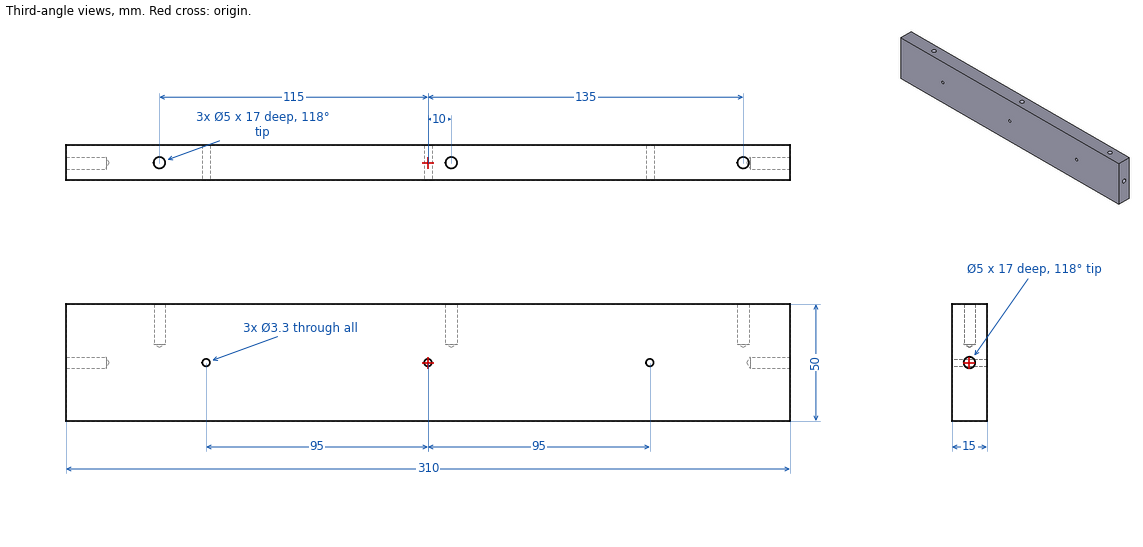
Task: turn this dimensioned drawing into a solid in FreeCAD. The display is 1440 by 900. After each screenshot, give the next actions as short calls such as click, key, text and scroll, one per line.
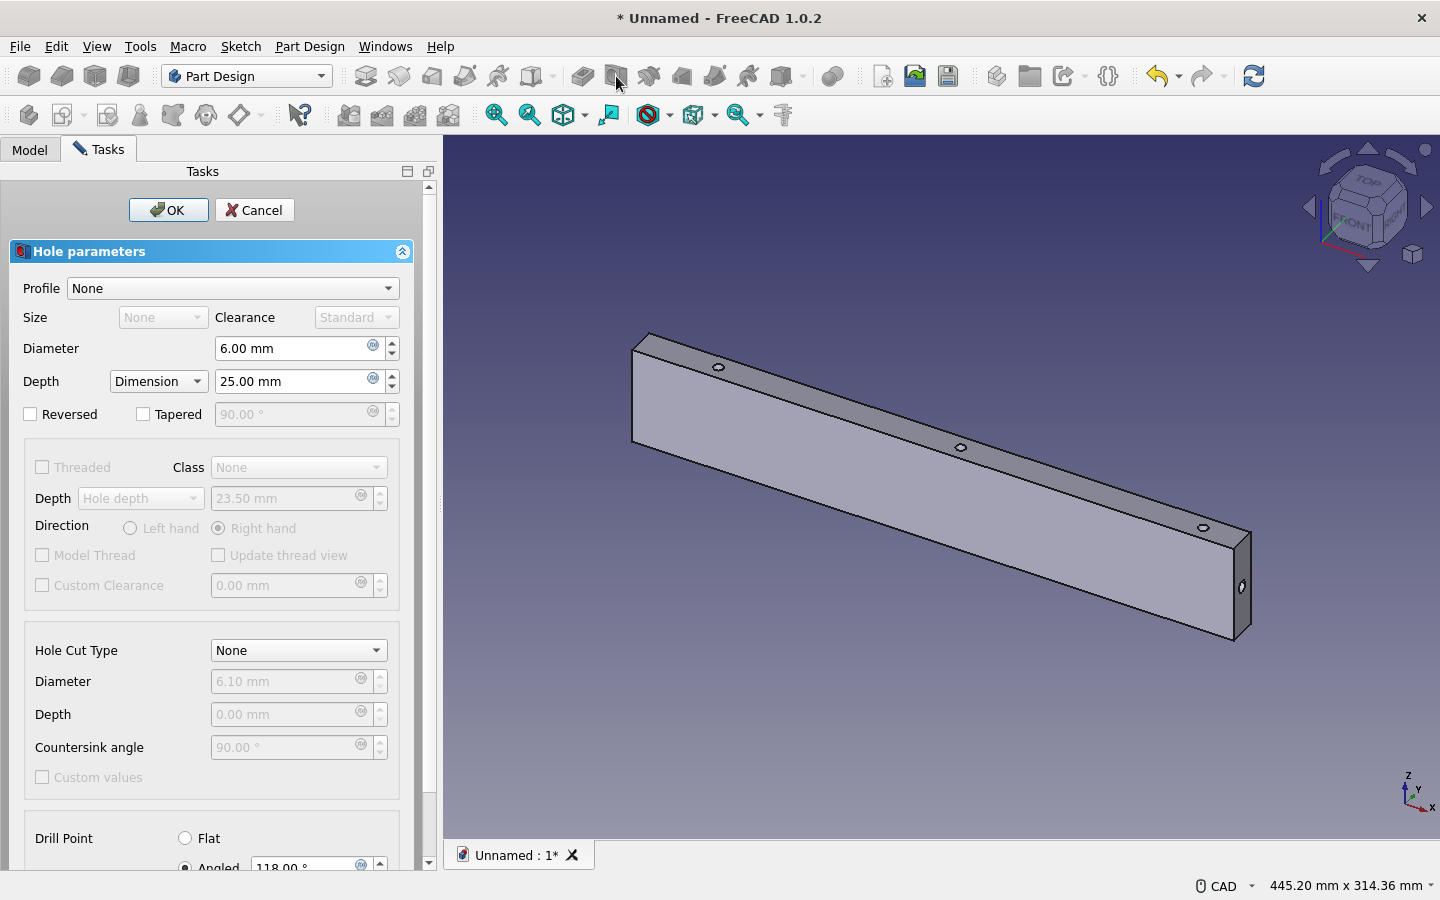
triple_click(300, 348)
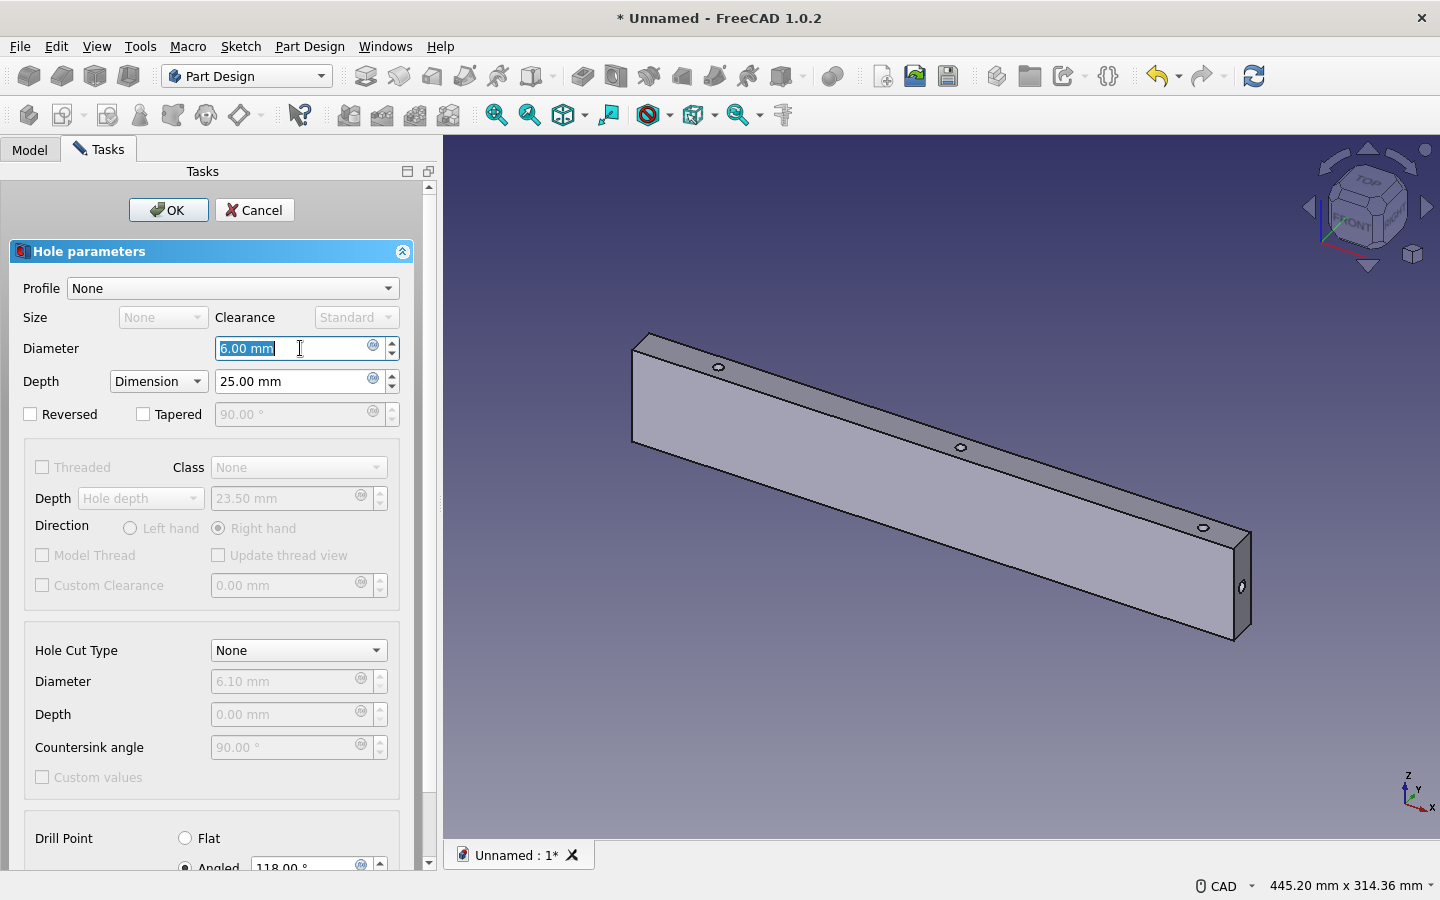
text(5)
key(Tab)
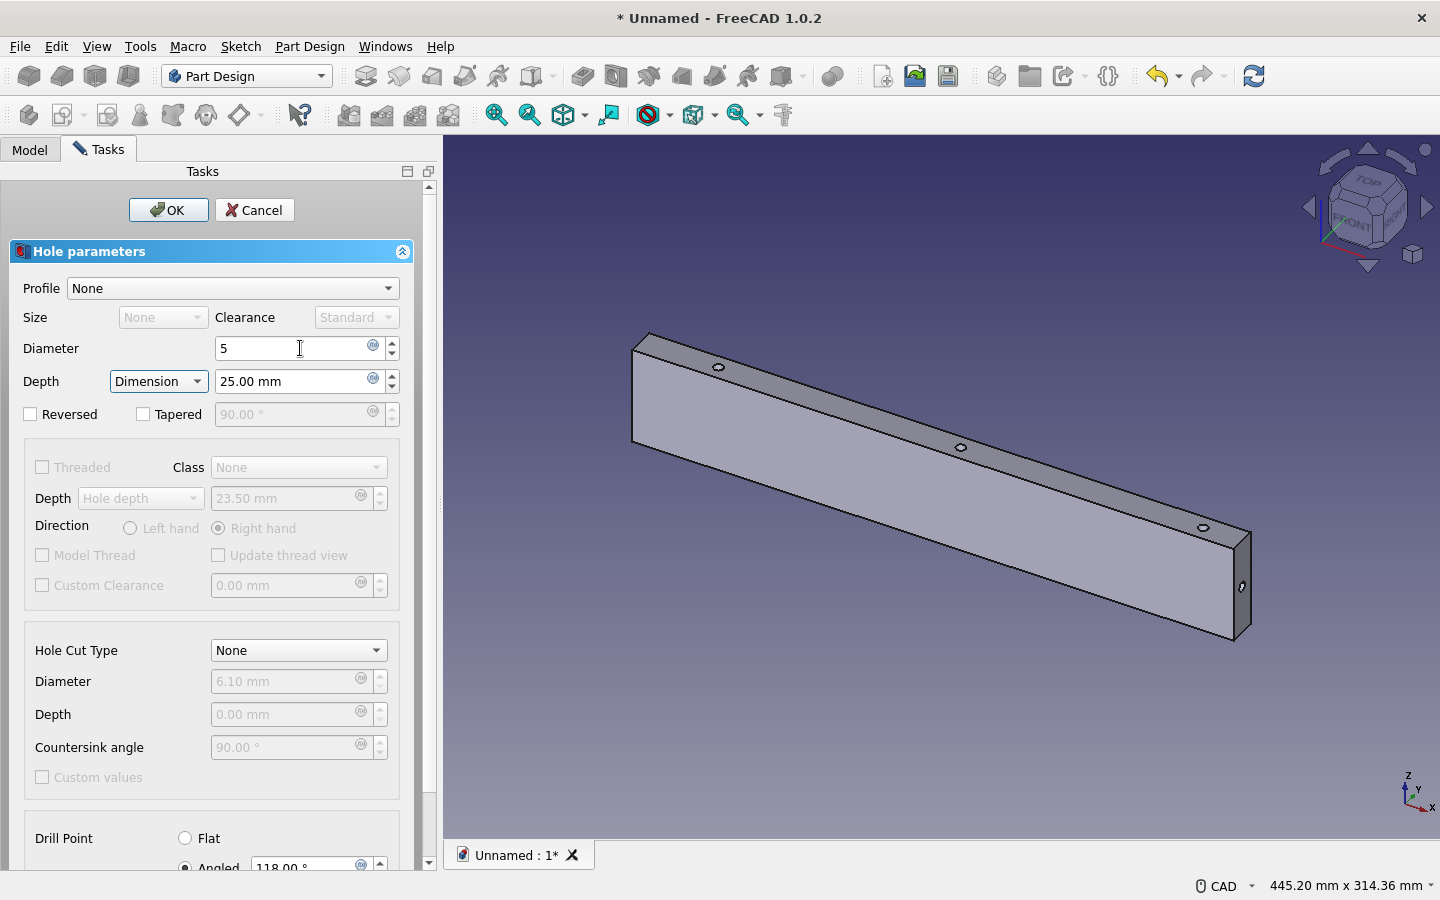
triple_click(300, 382)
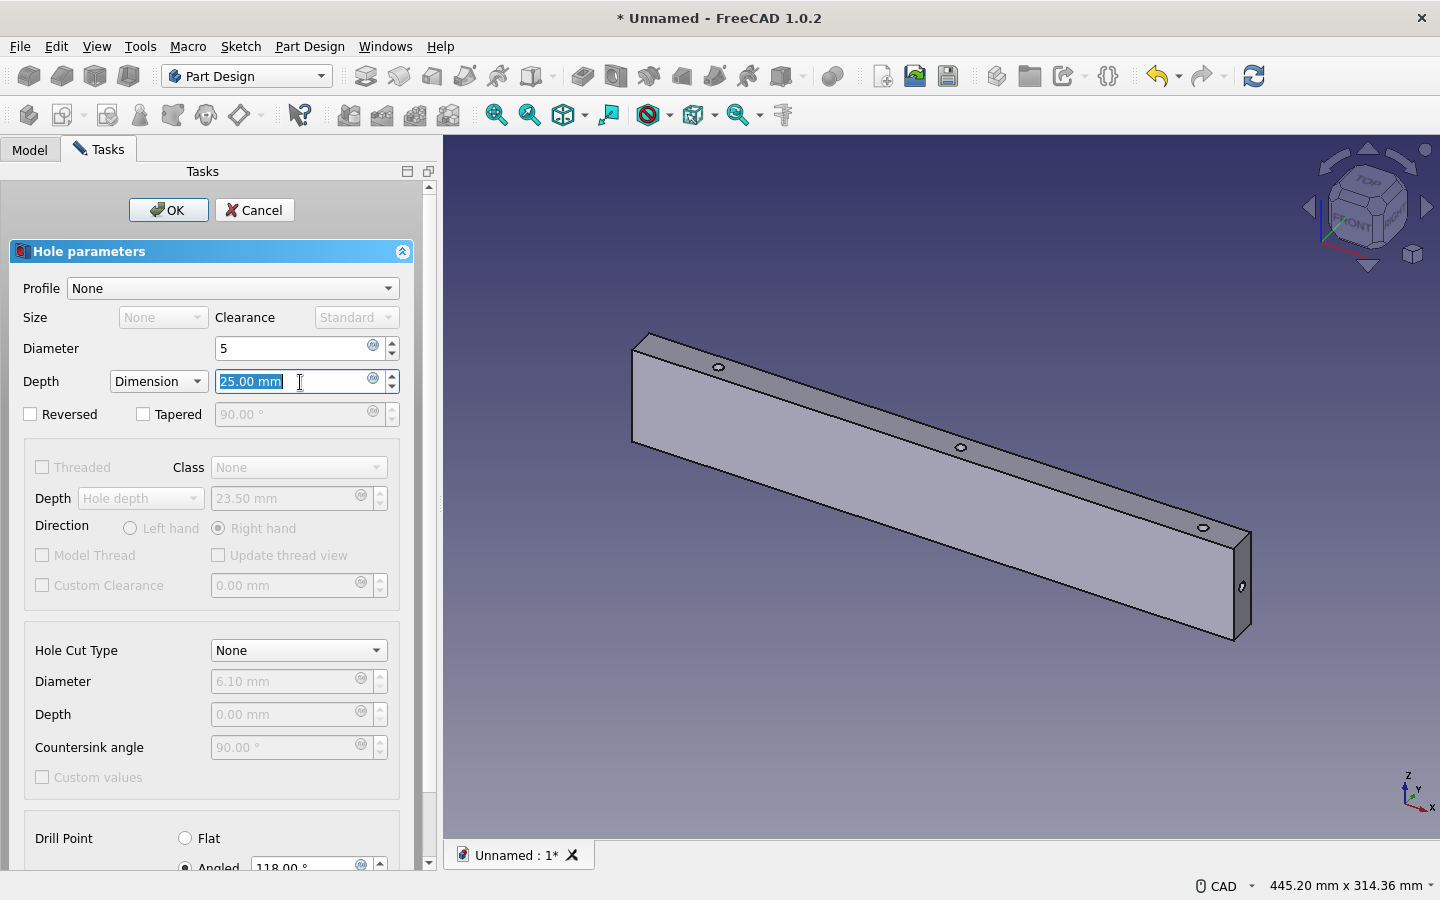
text(17)
key(Tab)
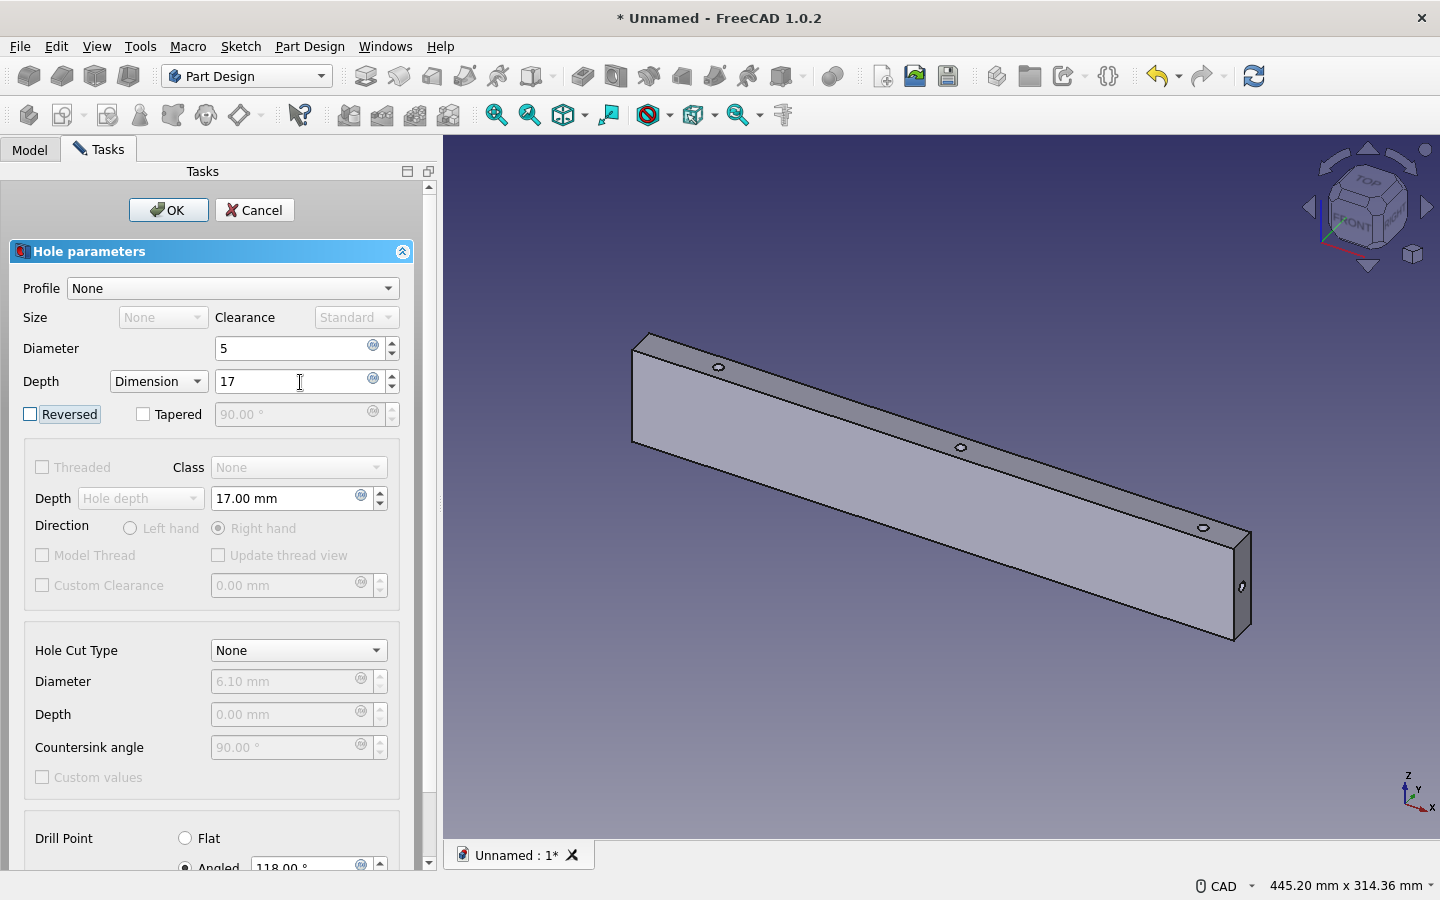
click(169, 210)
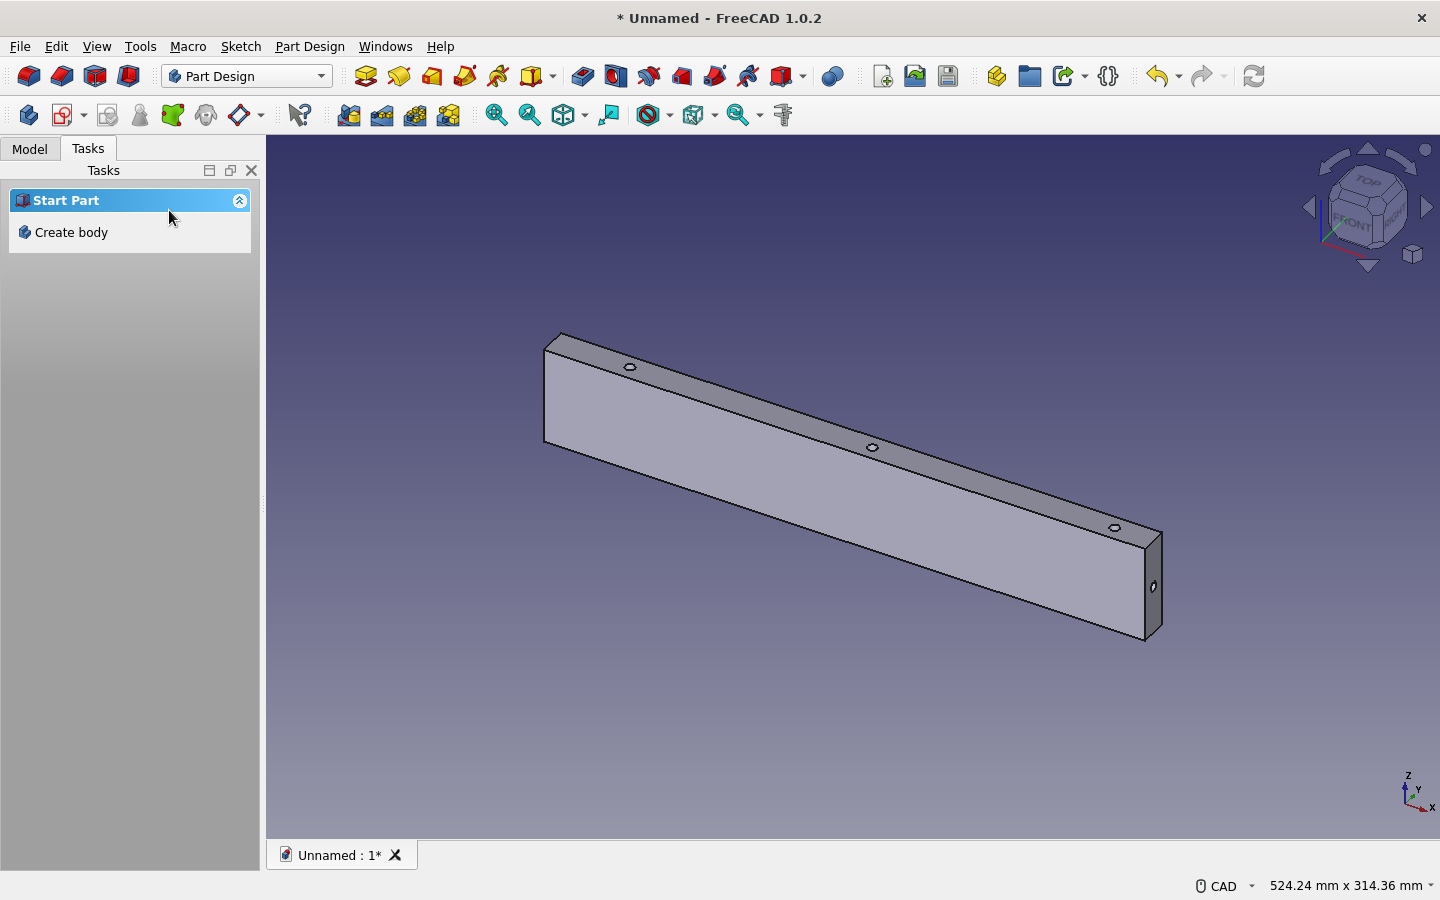
key(6)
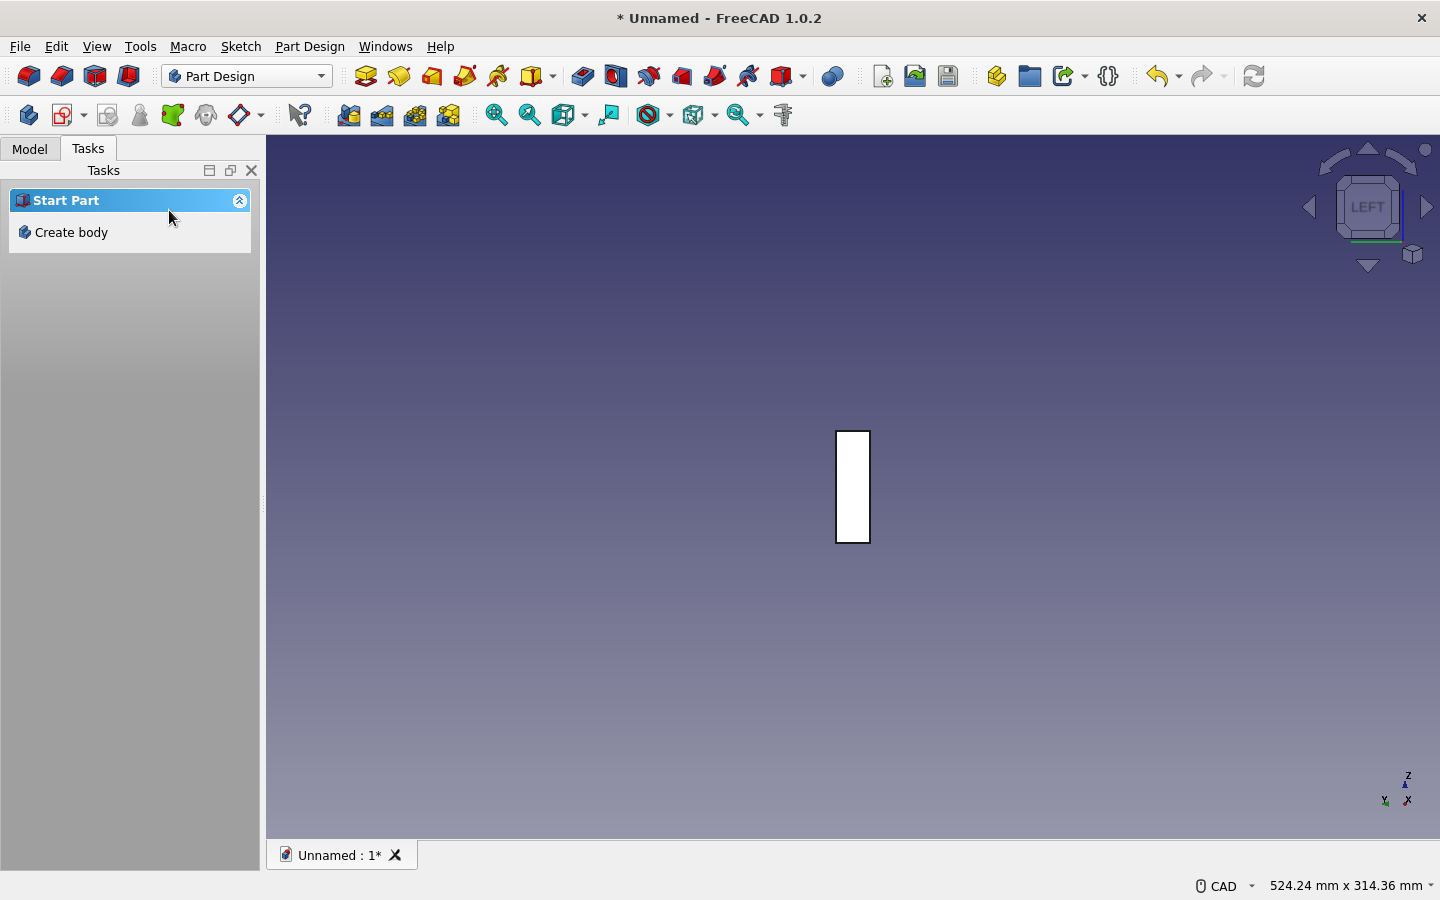
click(497, 116)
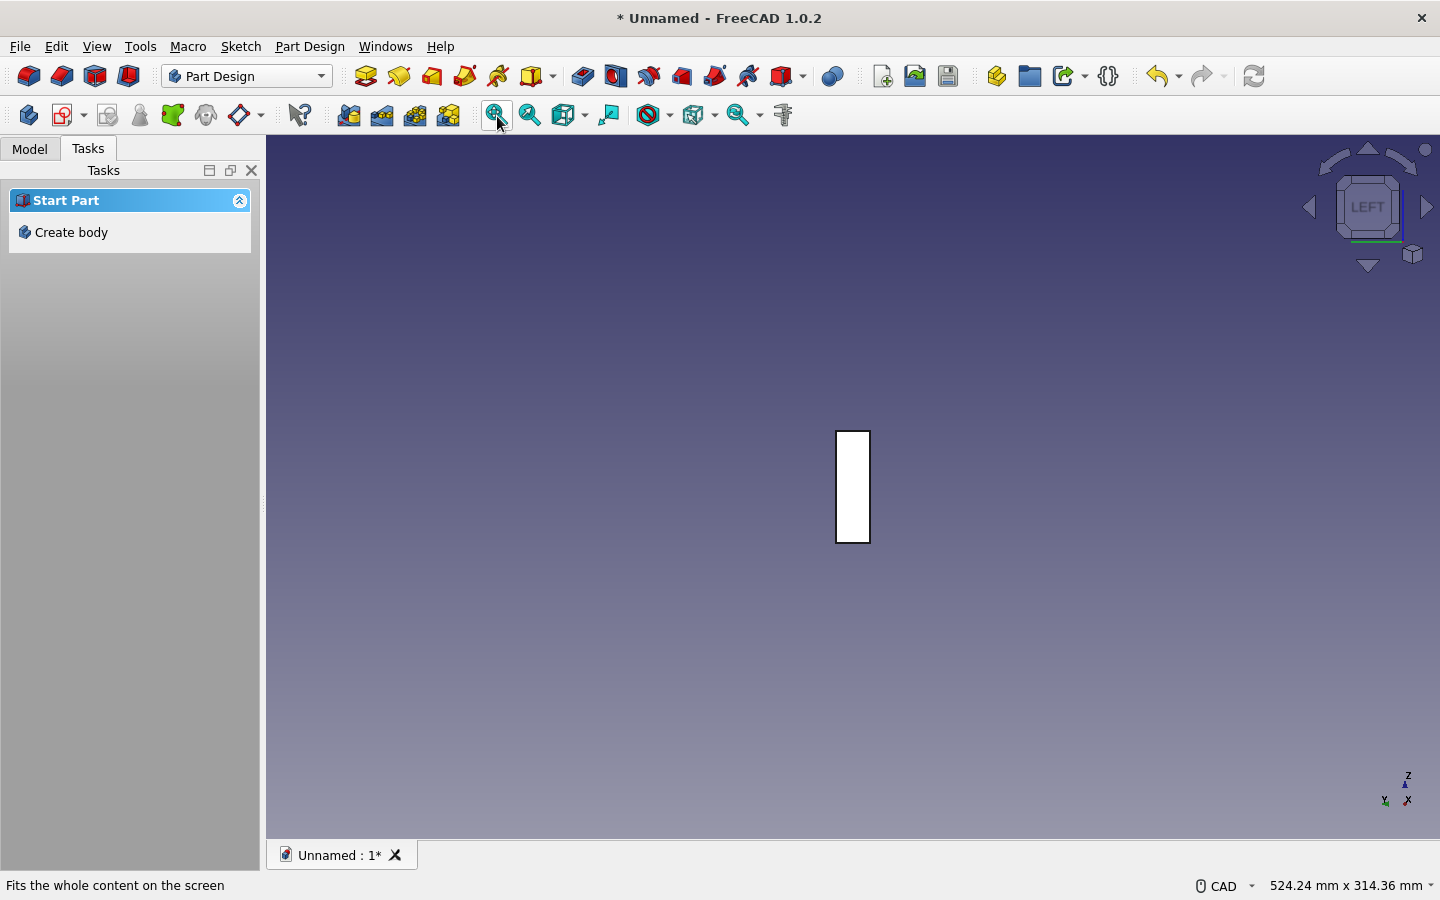
click(853, 454)